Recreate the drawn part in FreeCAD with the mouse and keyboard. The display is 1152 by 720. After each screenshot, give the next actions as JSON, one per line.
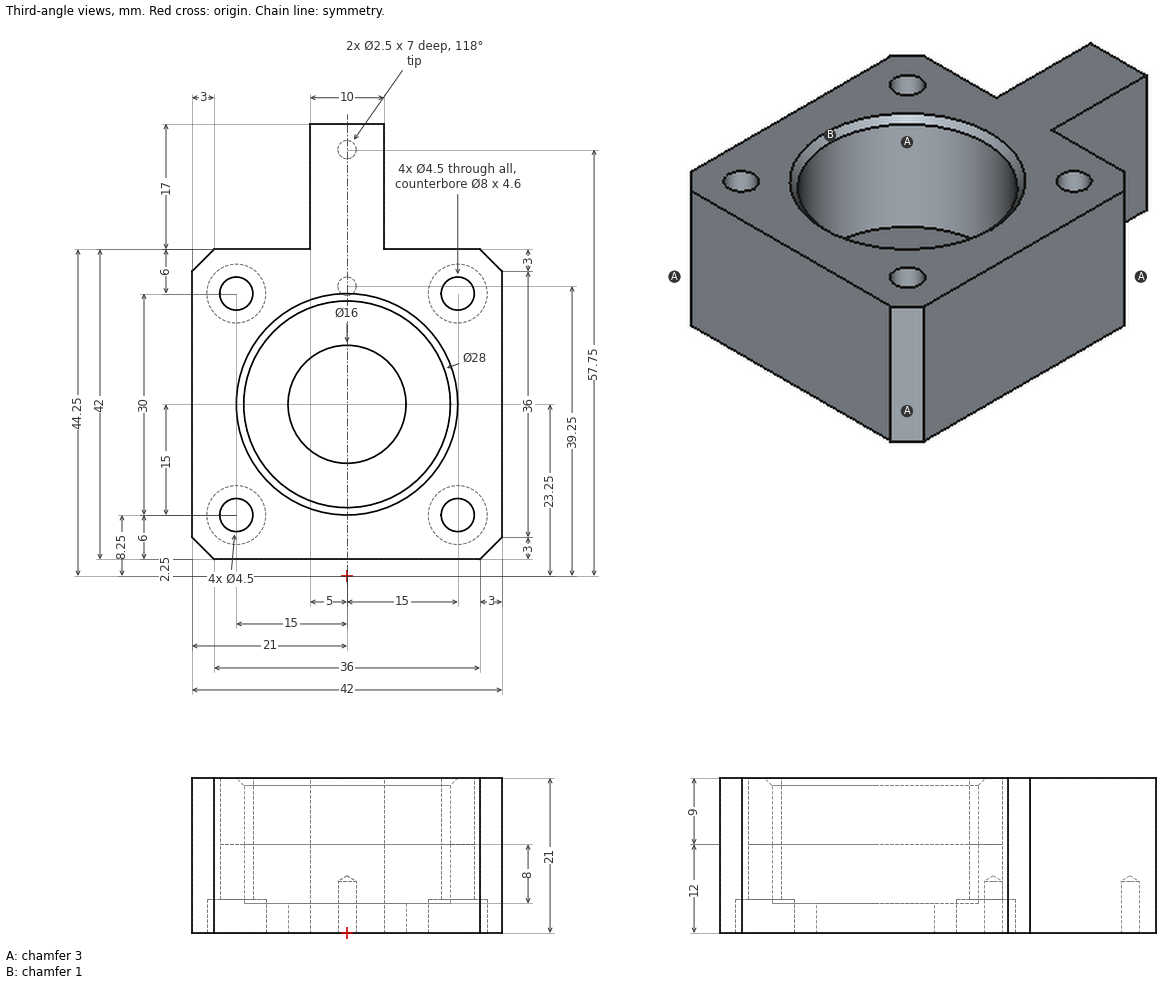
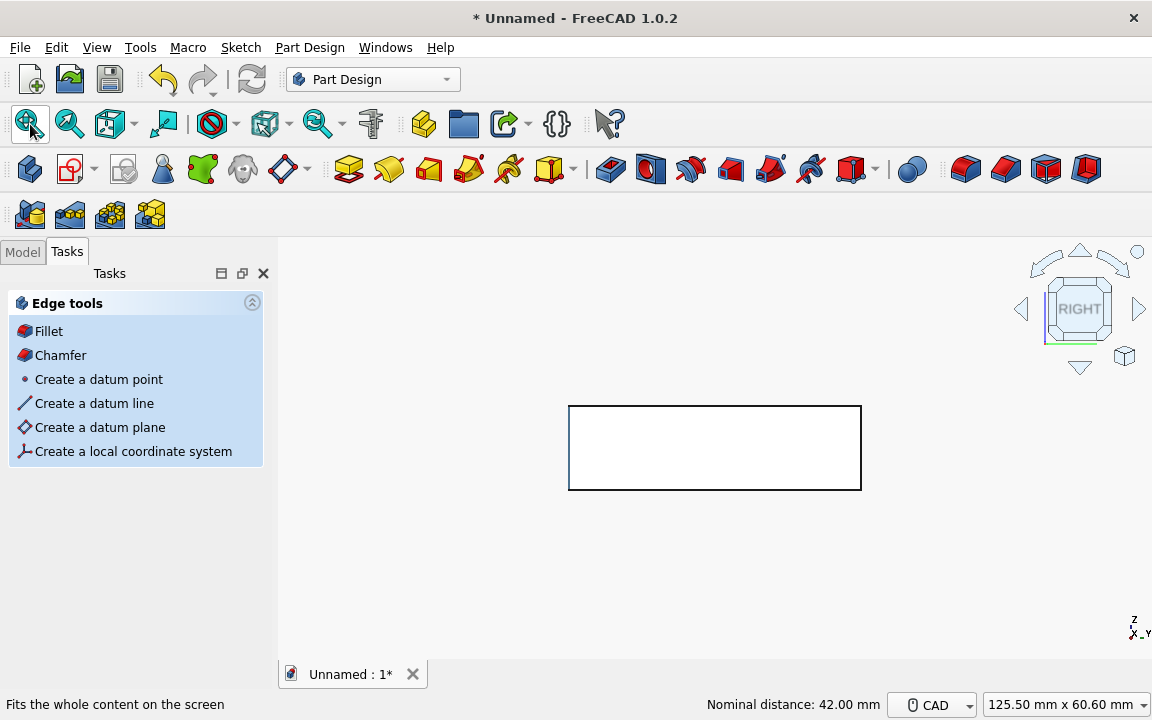
{"action": "left_click", "coordinate": [861, 447], "text": "ctrl"}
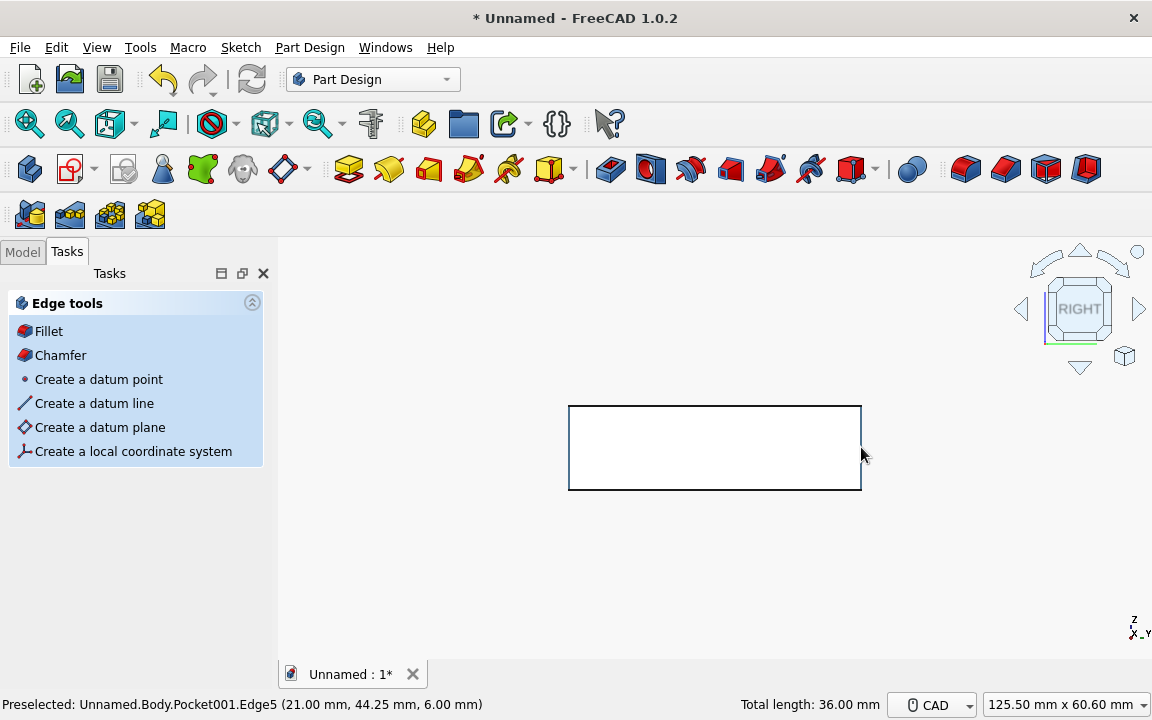
{"action": "key", "text": "5"}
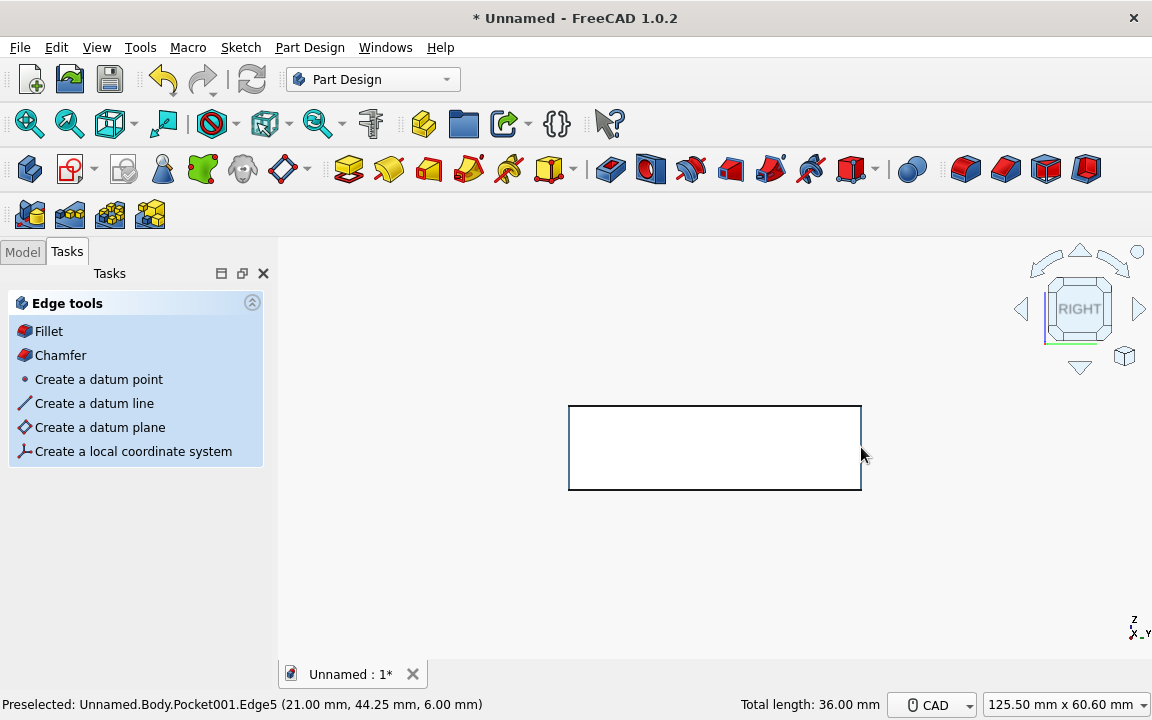
{"action": "key", "text": "4"}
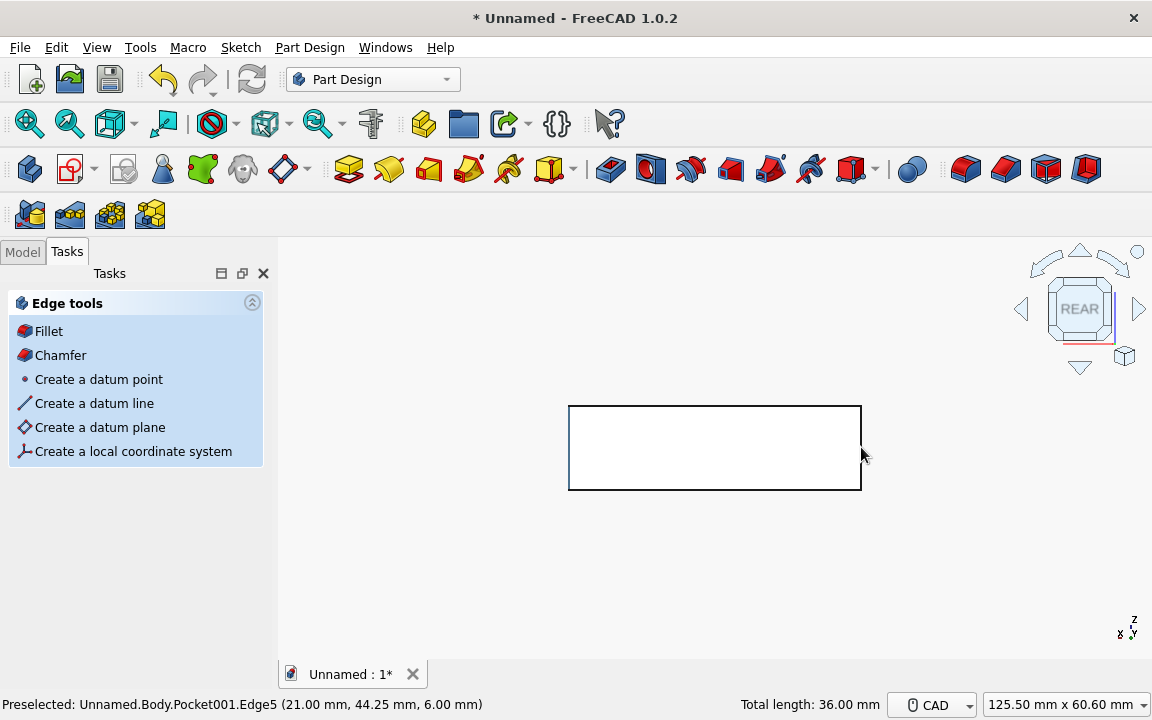
{"action": "left_click", "coordinate": [30, 124]}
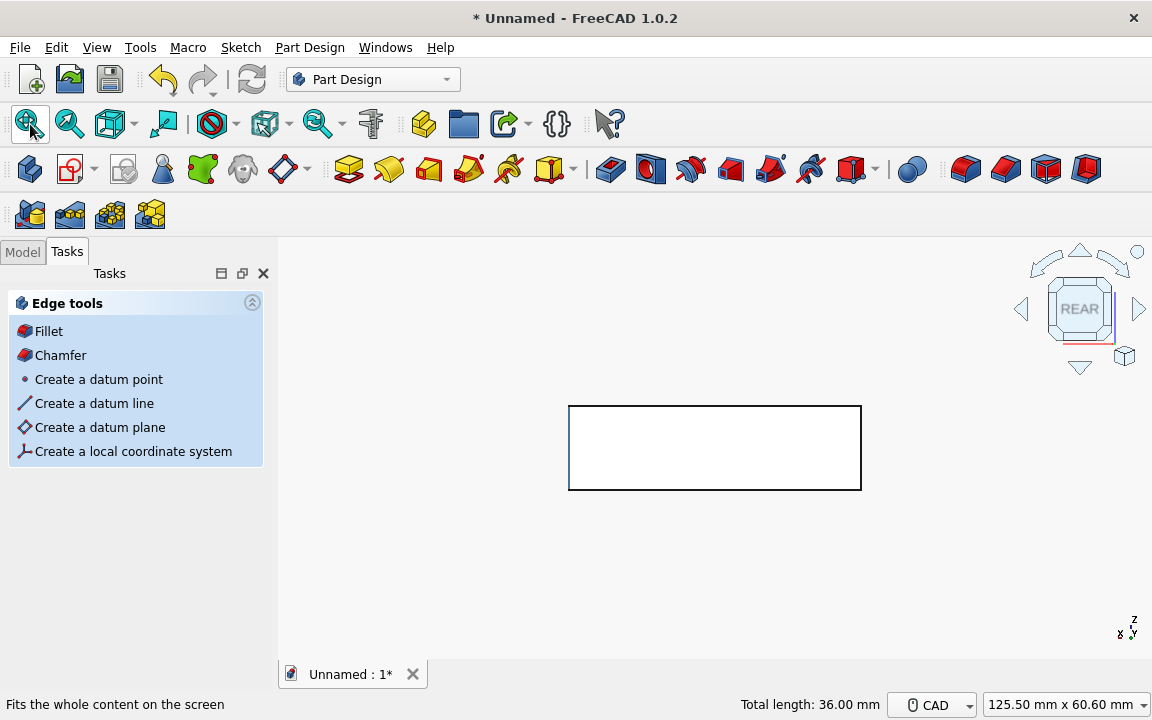
{"action": "left_click", "coordinate": [861, 447], "text": "ctrl"}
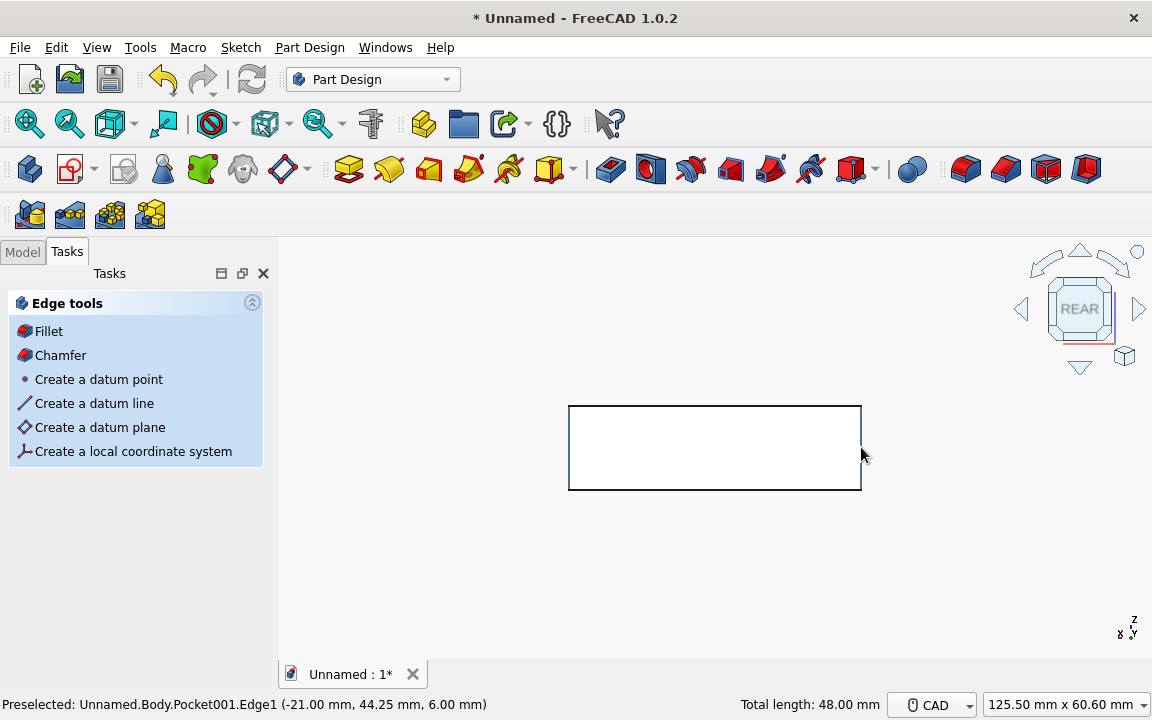
{"action": "left_click", "coordinate": [1006, 170]}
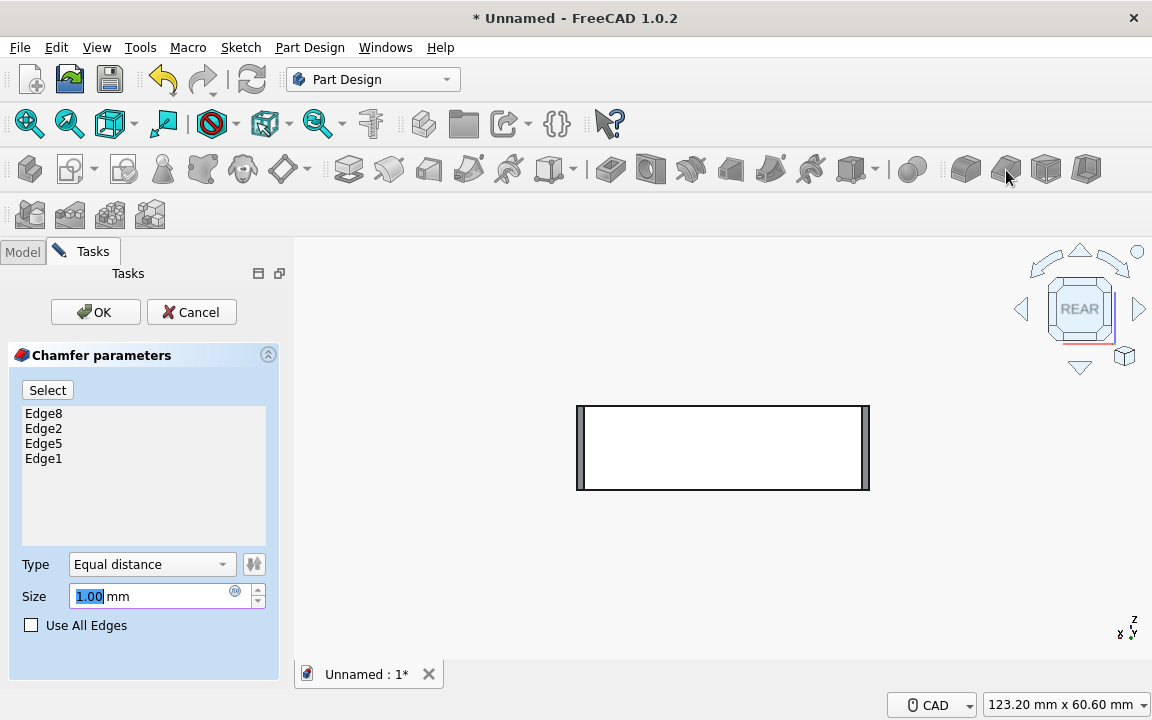
{"action": "type", "text": "3"}
{"action": "key", "text": "Tab"}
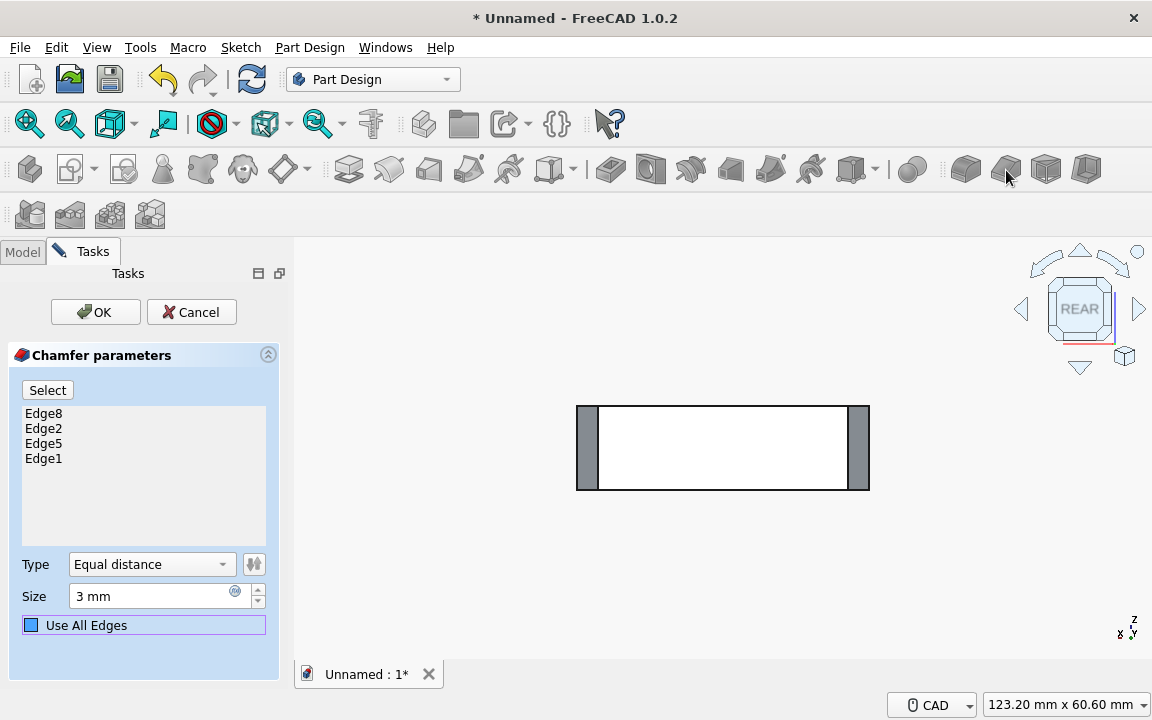
{"action": "left_click", "coordinate": [96, 312]}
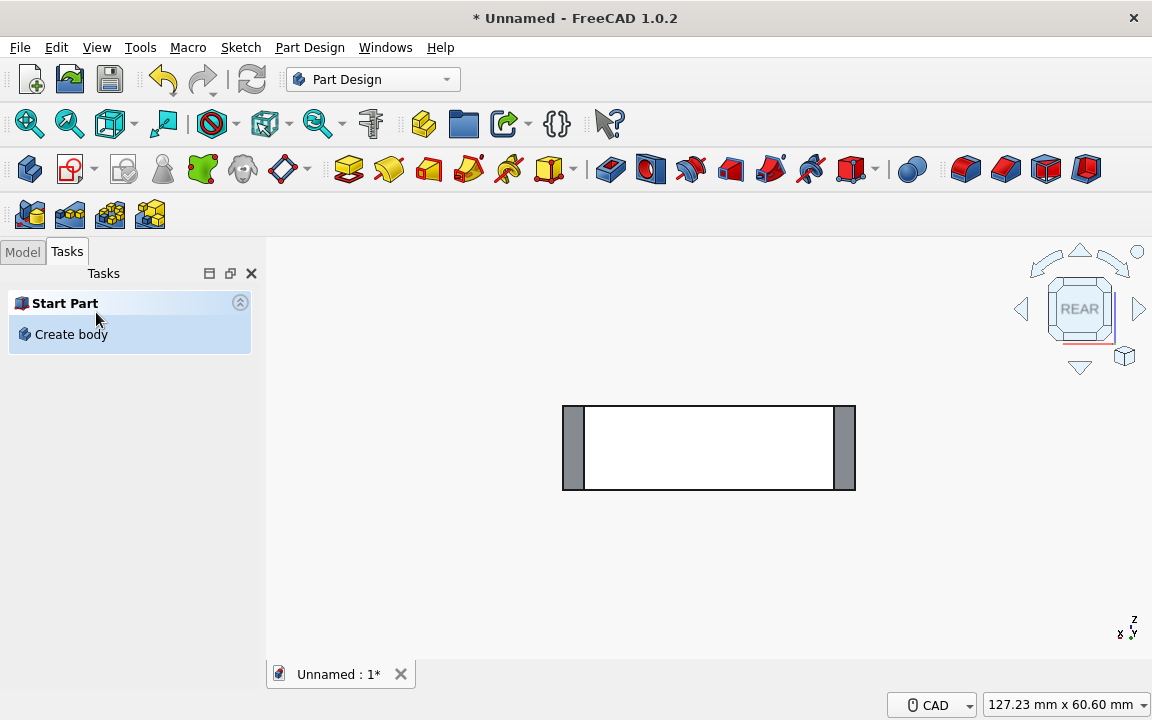
{"action": "left_click", "coordinate": [30, 124]}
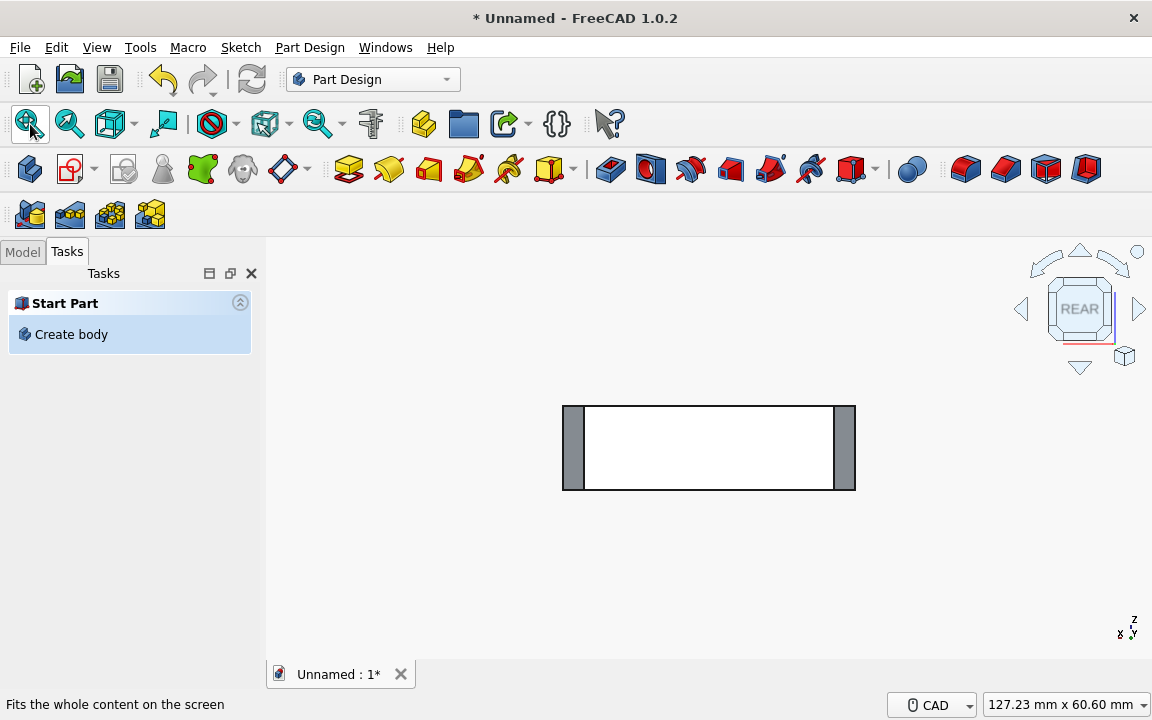
{"action": "key", "text": "5"}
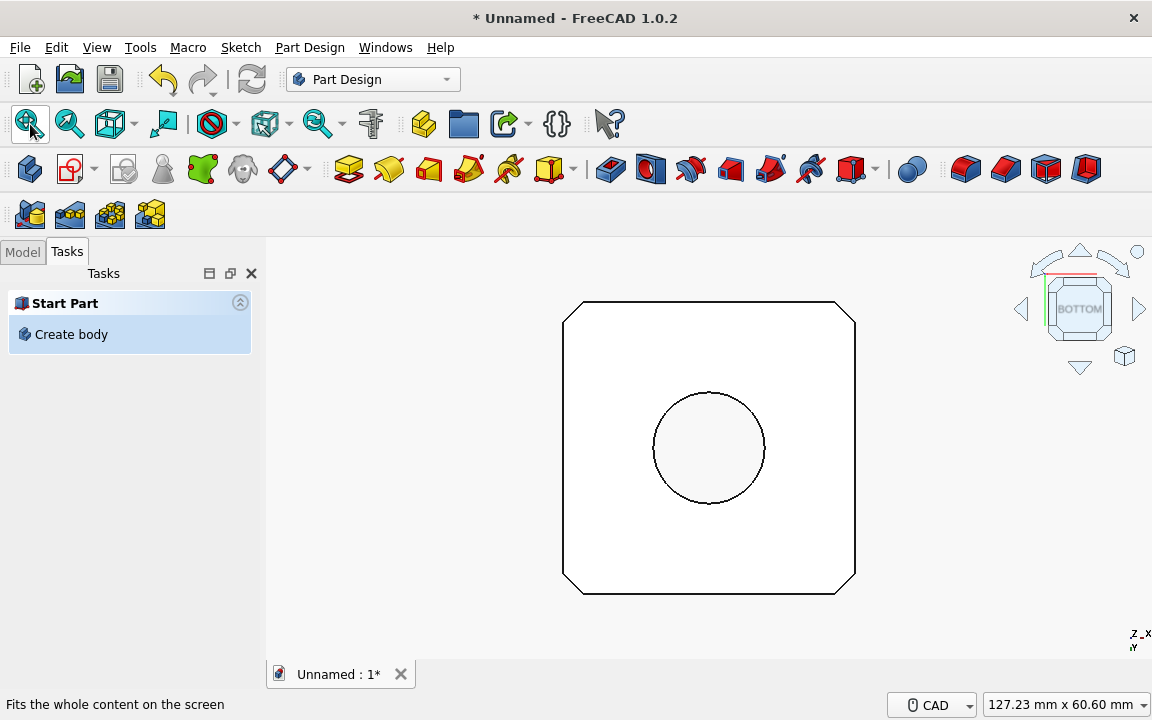
{"action": "left_click", "coordinate": [793, 531]}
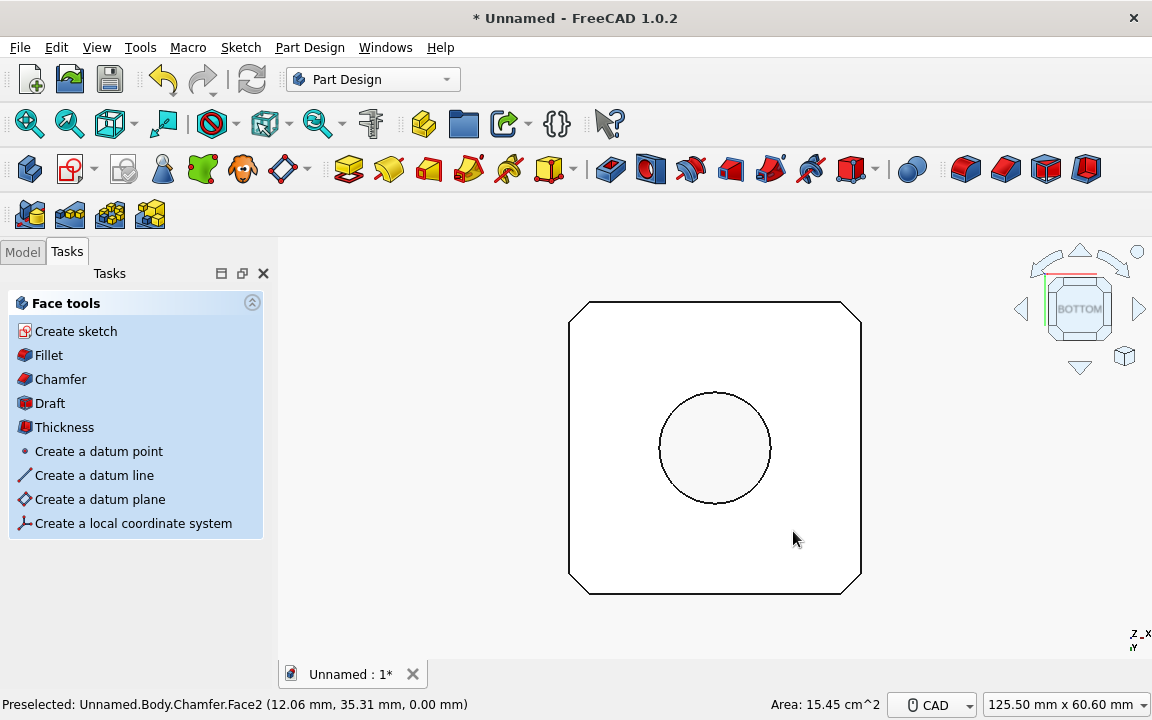
{"action": "left_click", "coordinate": [70, 170]}